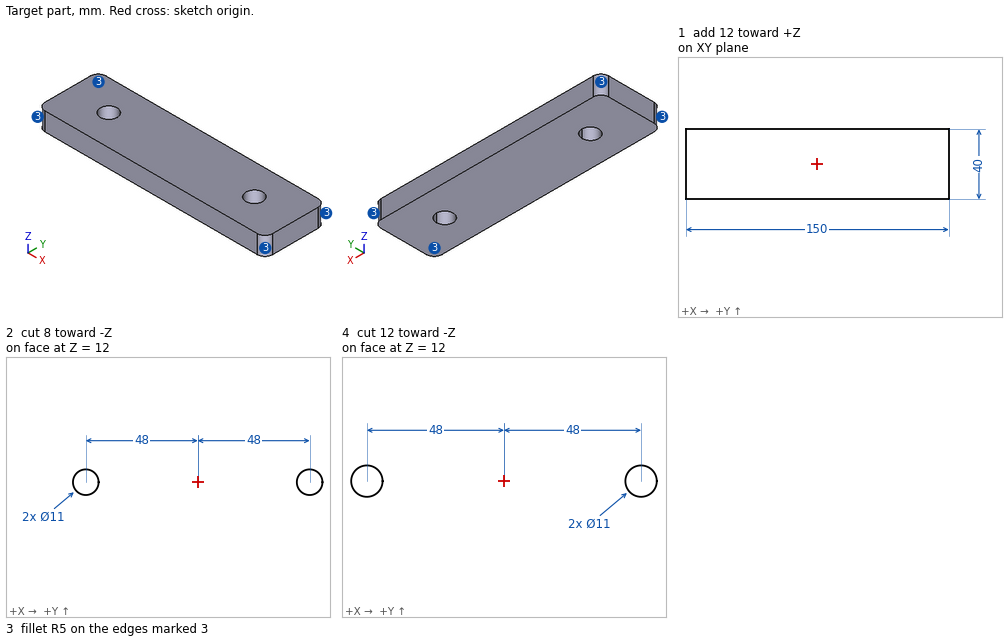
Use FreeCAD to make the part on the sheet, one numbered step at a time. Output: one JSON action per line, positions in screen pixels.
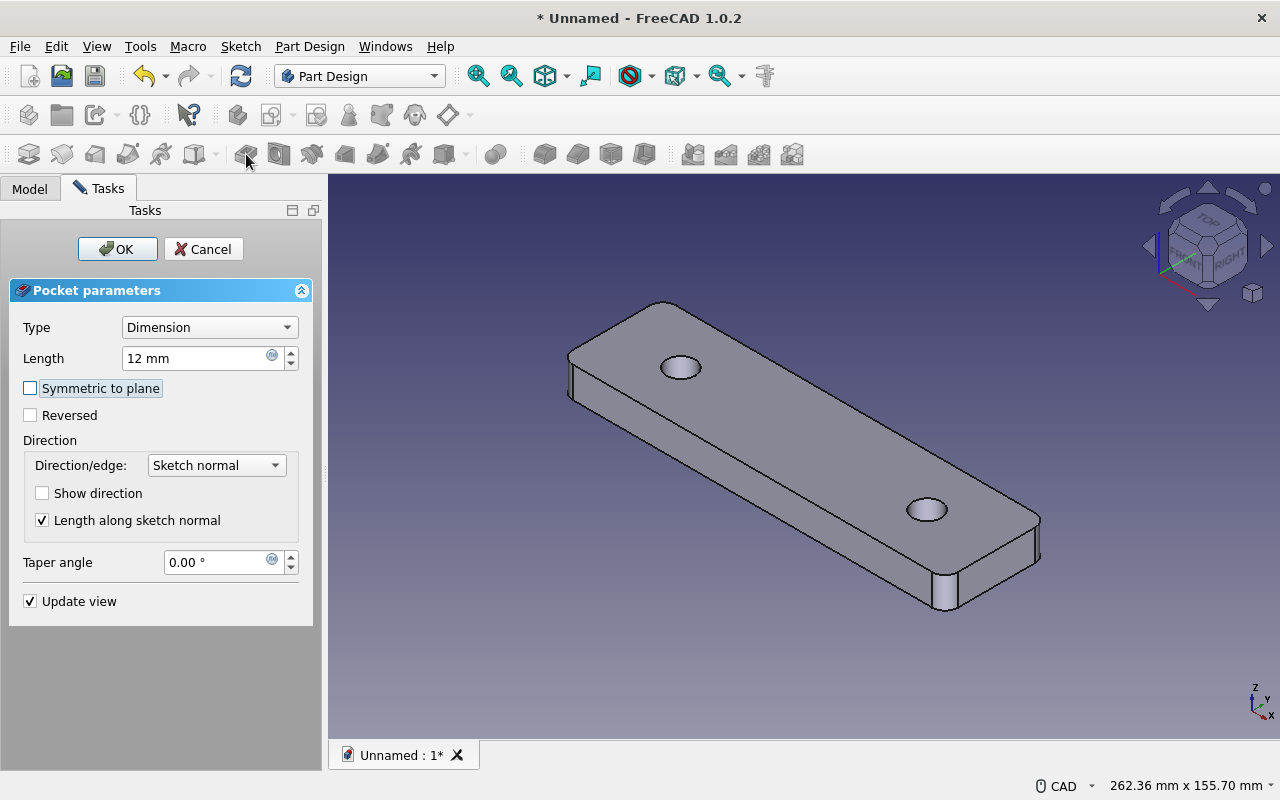
{"action": "left_click", "coordinate": [118, 249]}